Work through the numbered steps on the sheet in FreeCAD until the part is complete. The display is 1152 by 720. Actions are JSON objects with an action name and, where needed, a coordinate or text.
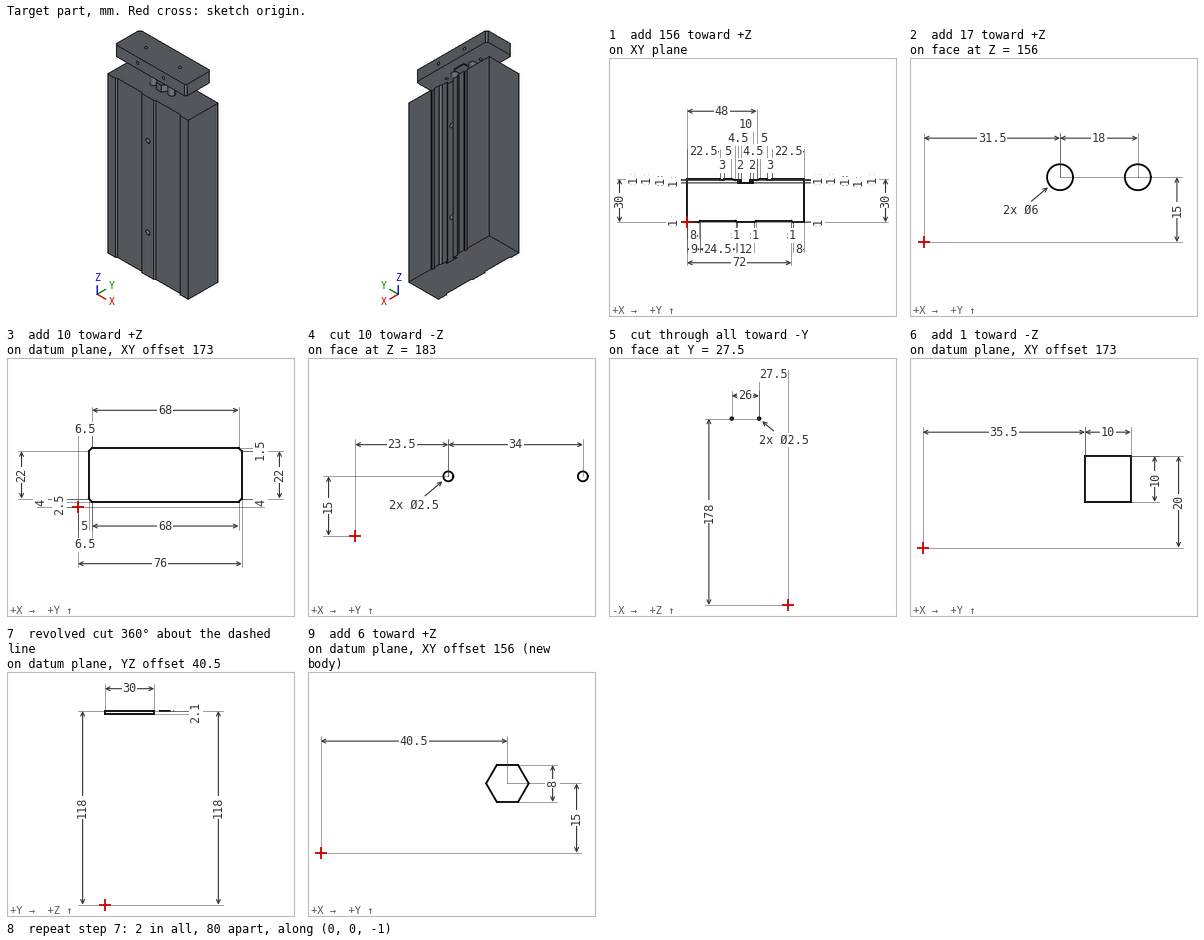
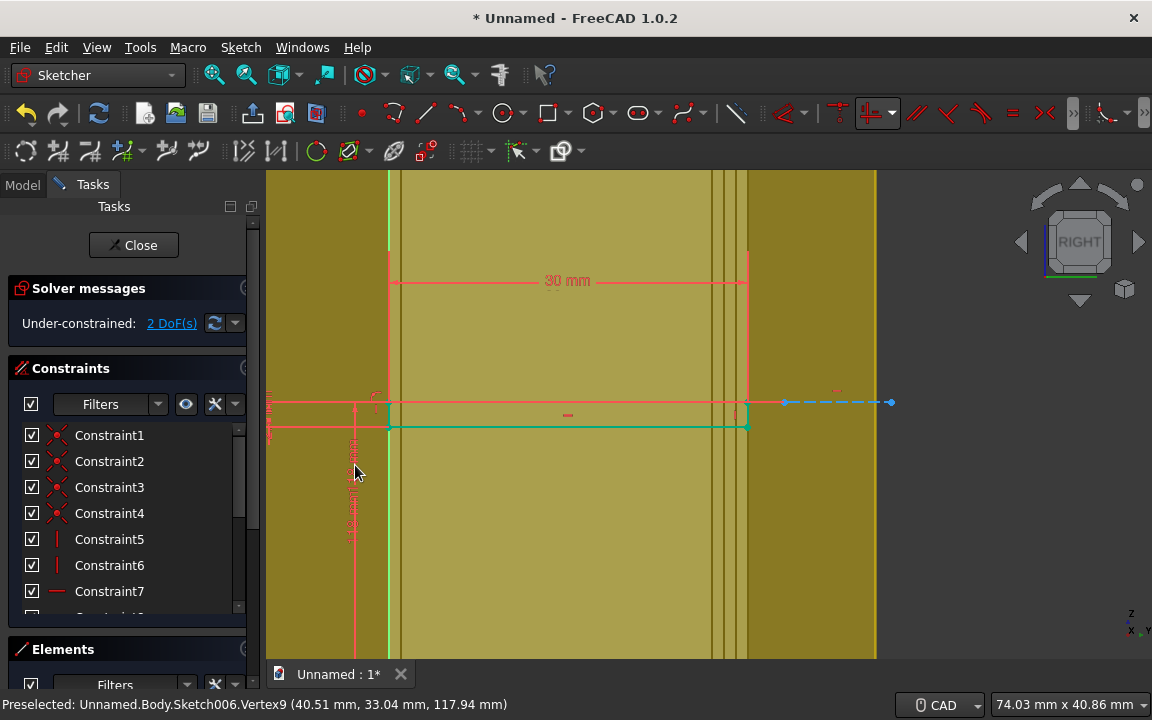
{"action": "left_click", "coordinate": [134, 245]}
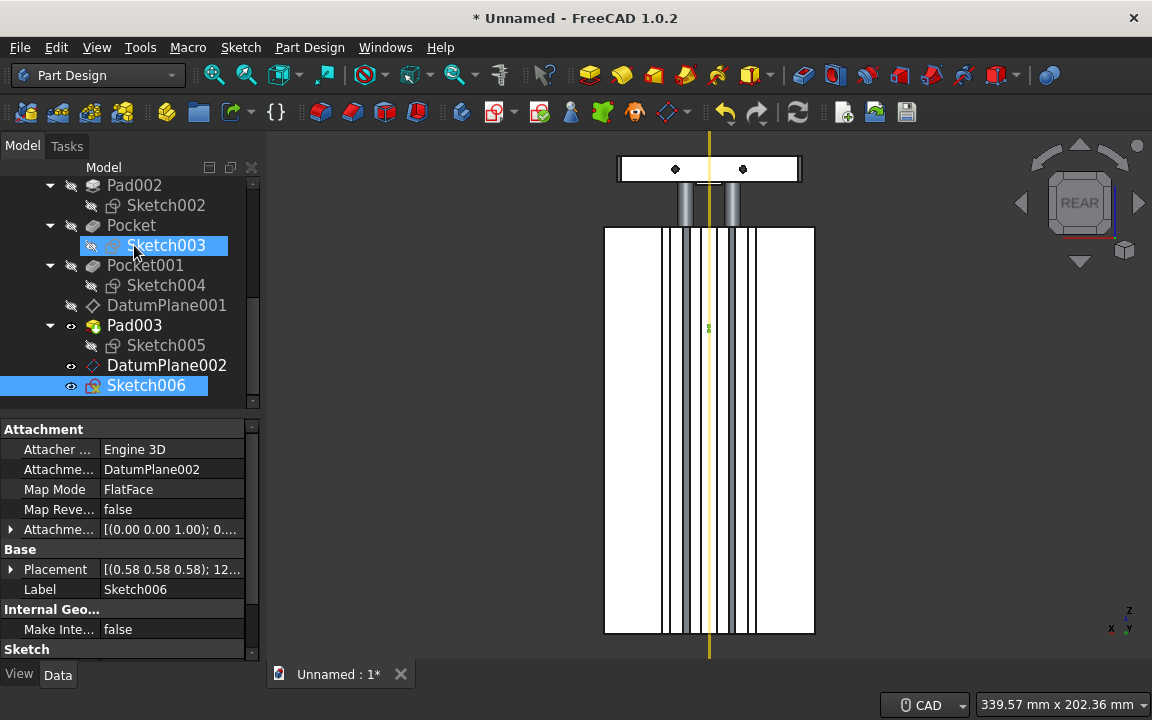
{"action": "left_click", "coordinate": [868, 76]}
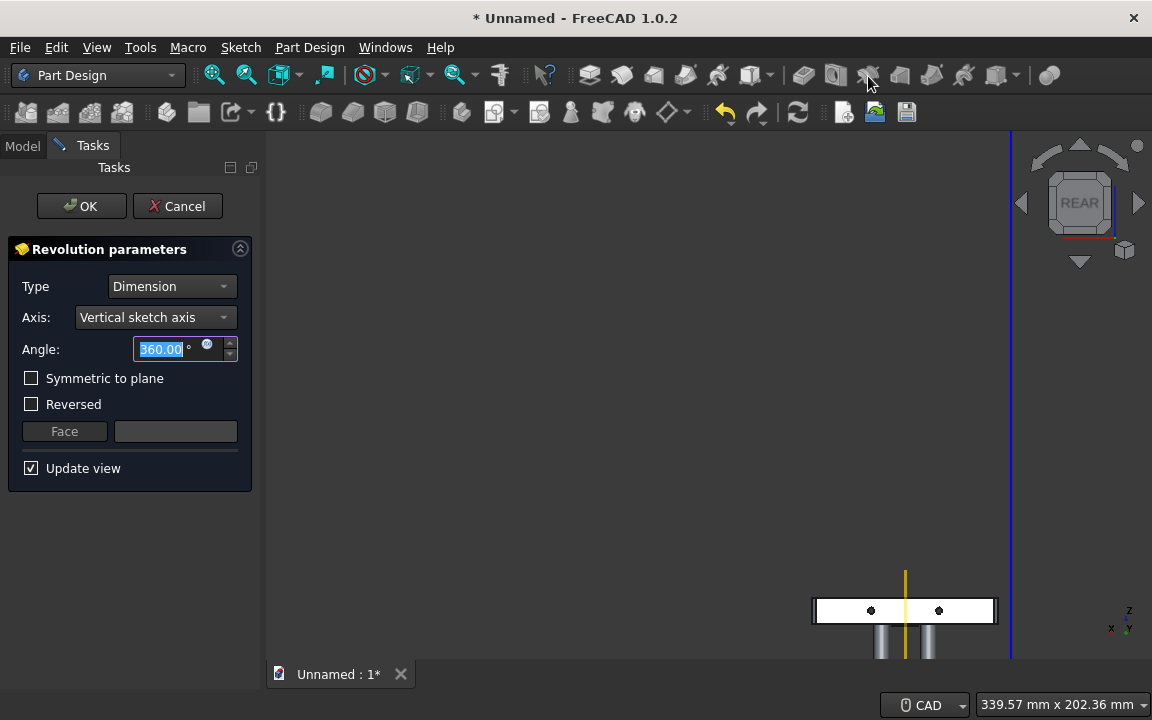
{"action": "left_click", "coordinate": [156, 318]}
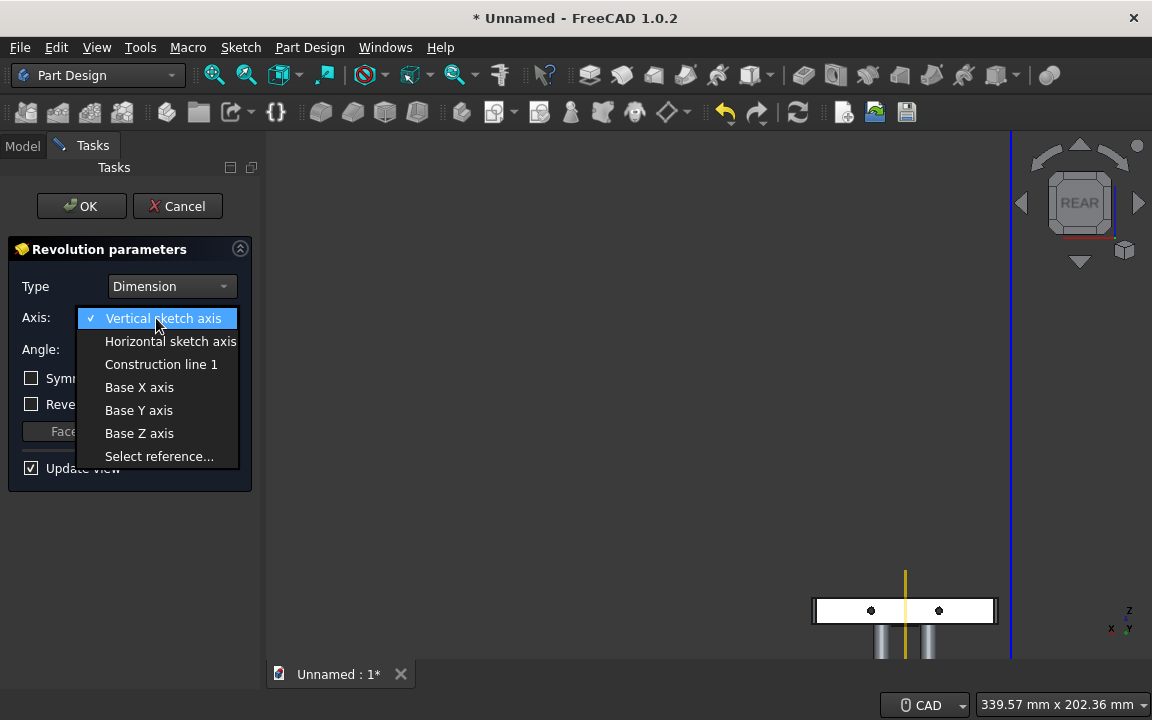
{"action": "left_click", "coordinate": [156, 364]}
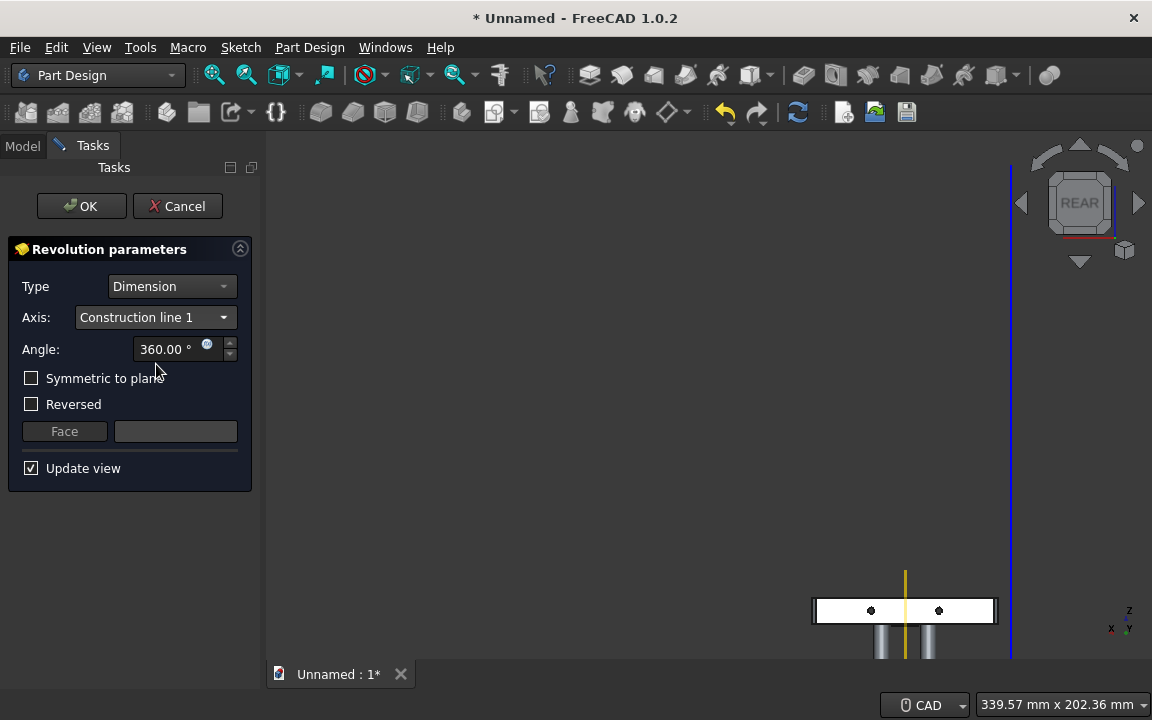
{"action": "left_click", "coordinate": [82, 206]}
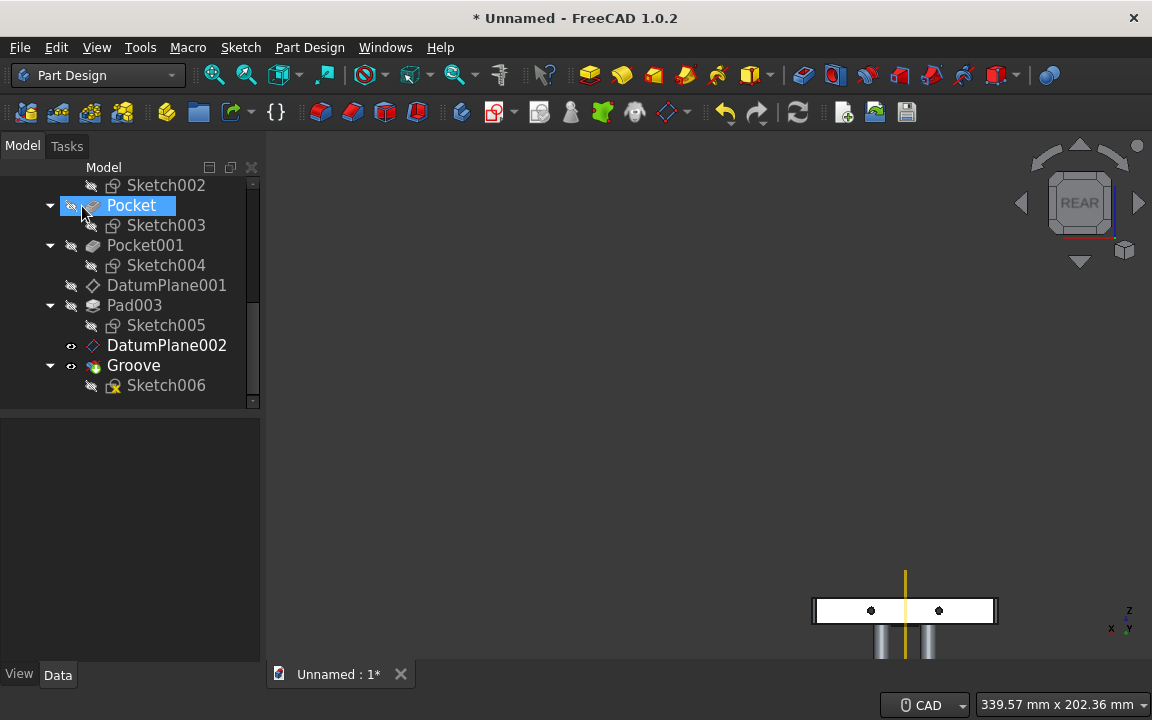
{"action": "left_click", "coordinate": [116, 346]}
{"action": "key", "text": "space"}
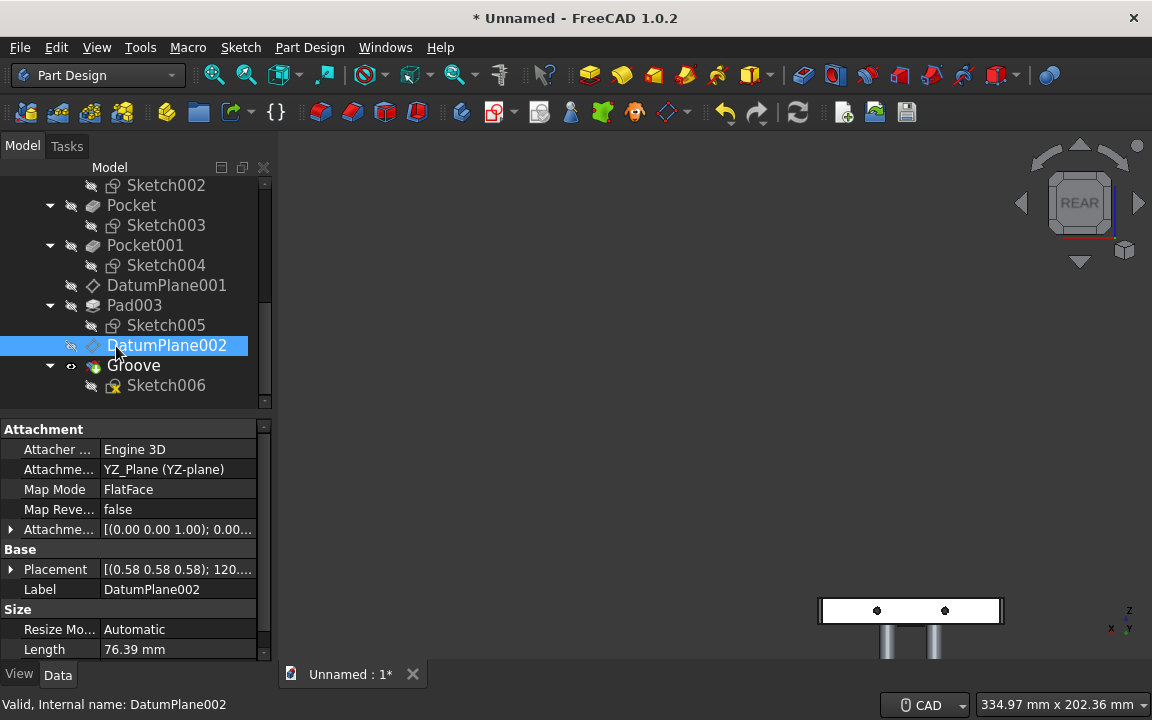
{"action": "key", "text": "v f"}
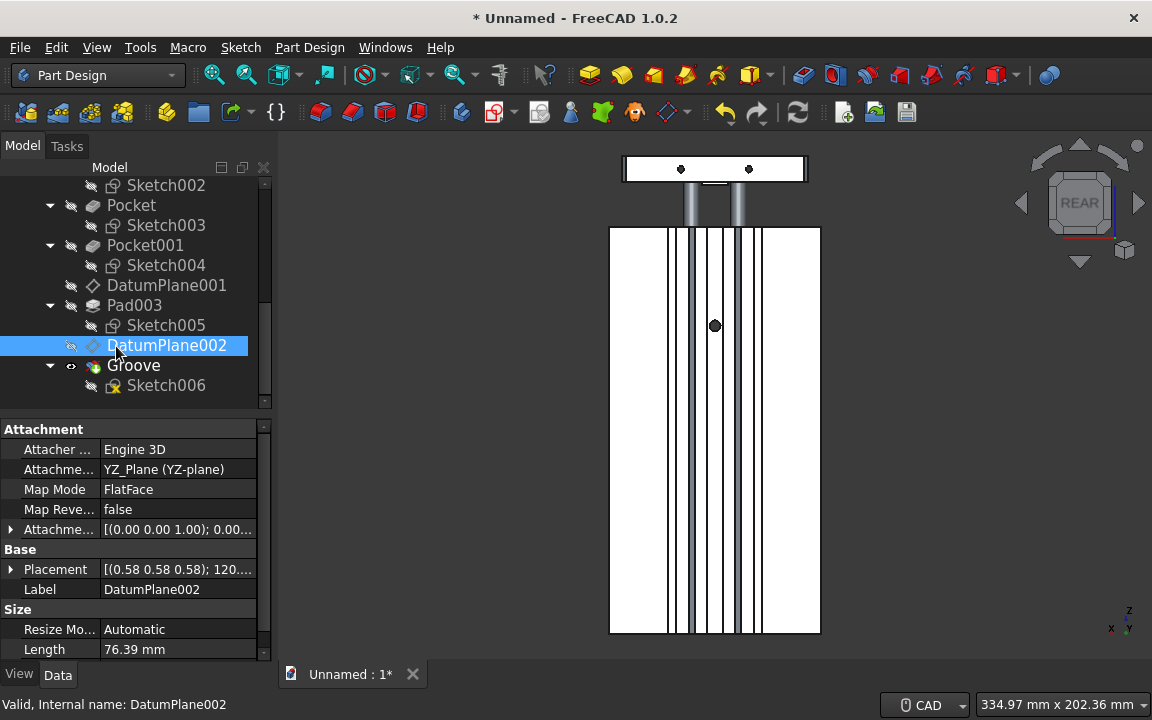
{"action": "left_click", "coordinate": [116, 366]}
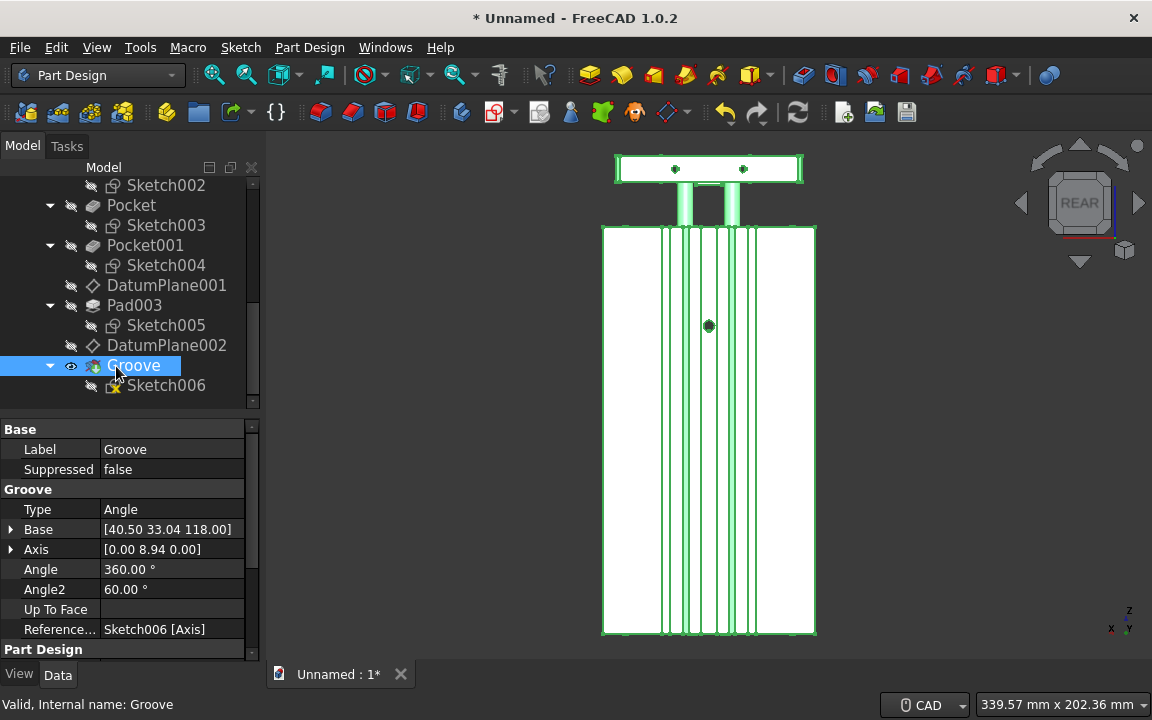
{"action": "left_click", "coordinate": [58, 112]}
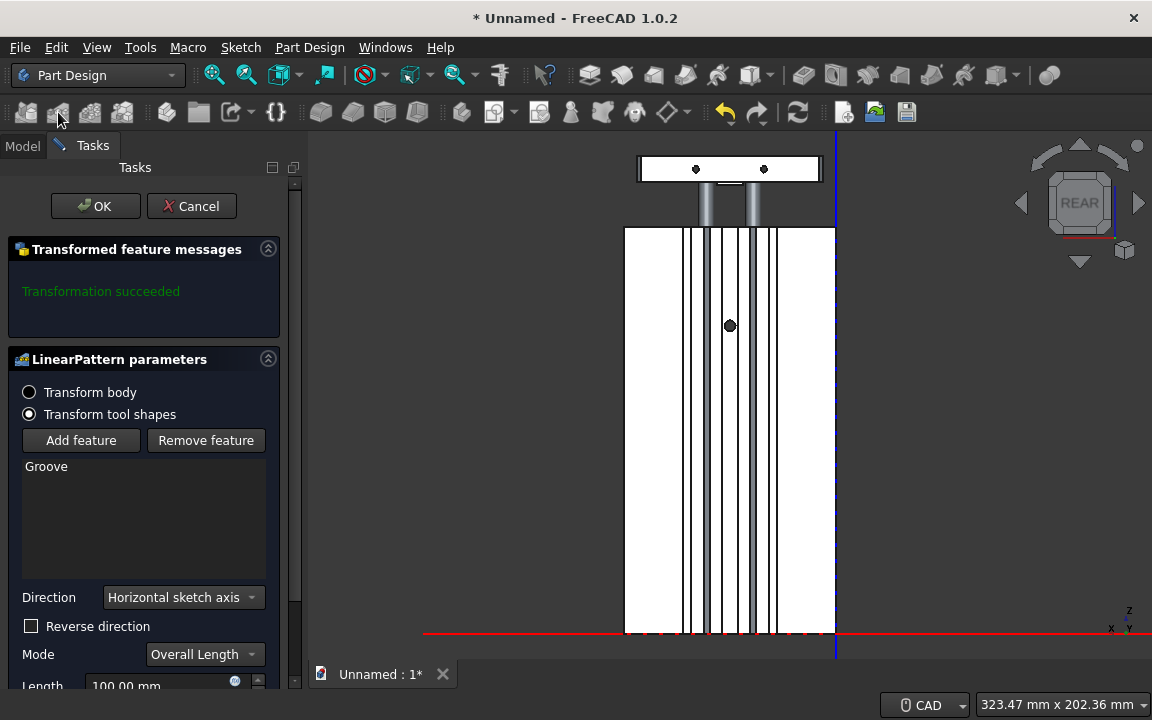
{"action": "left_click", "coordinate": [184, 598]}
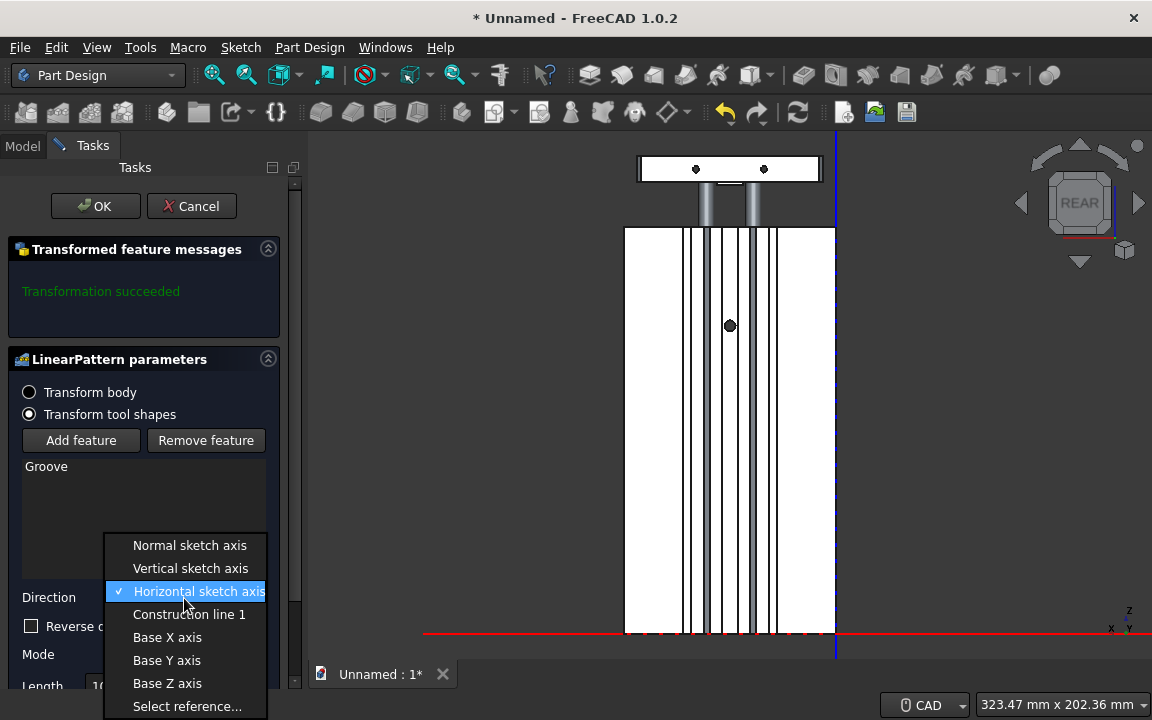
{"action": "left_click", "coordinate": [184, 684]}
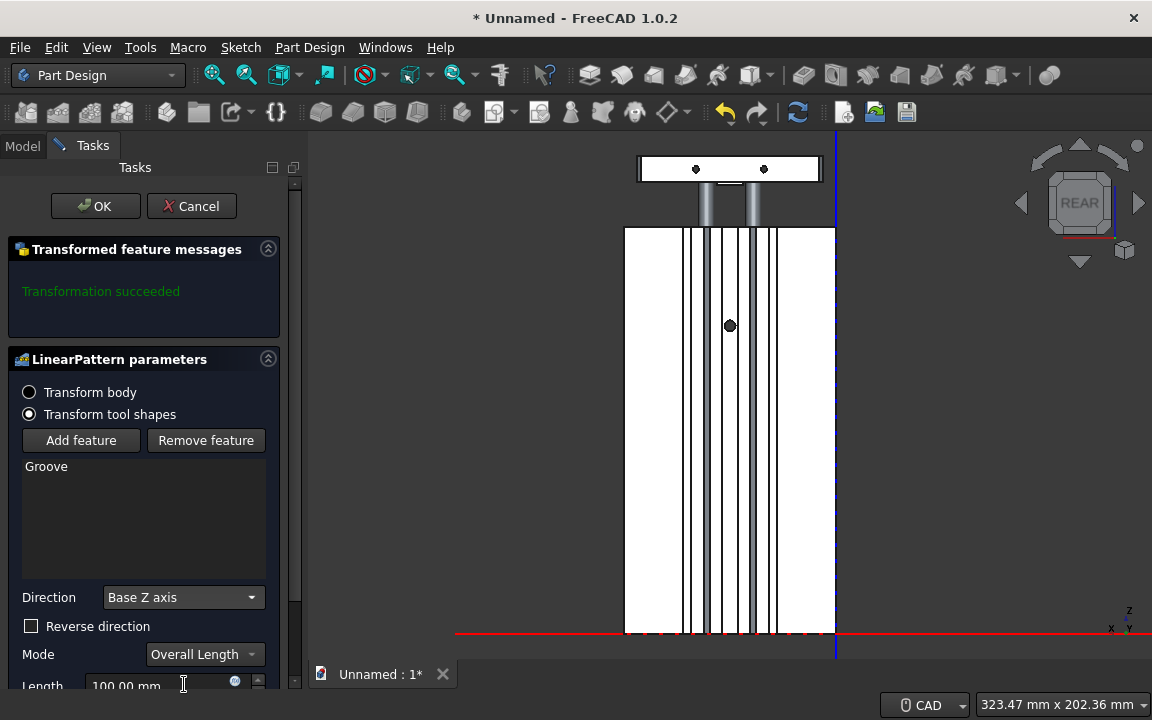
{"action": "left_click", "coordinate": [206, 654]}